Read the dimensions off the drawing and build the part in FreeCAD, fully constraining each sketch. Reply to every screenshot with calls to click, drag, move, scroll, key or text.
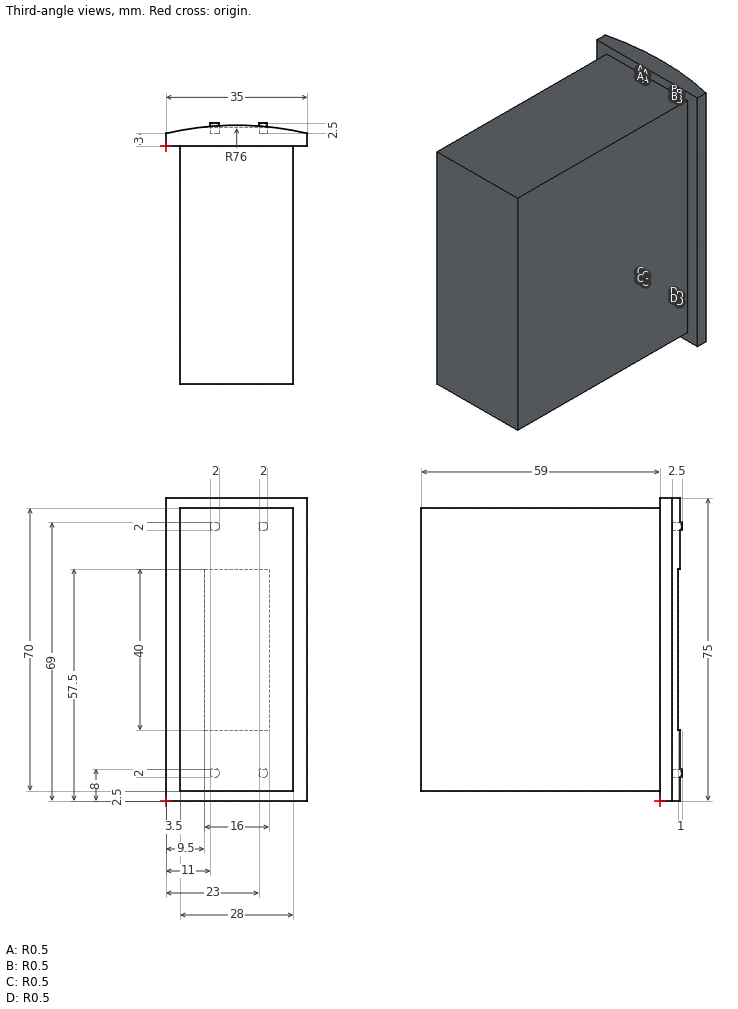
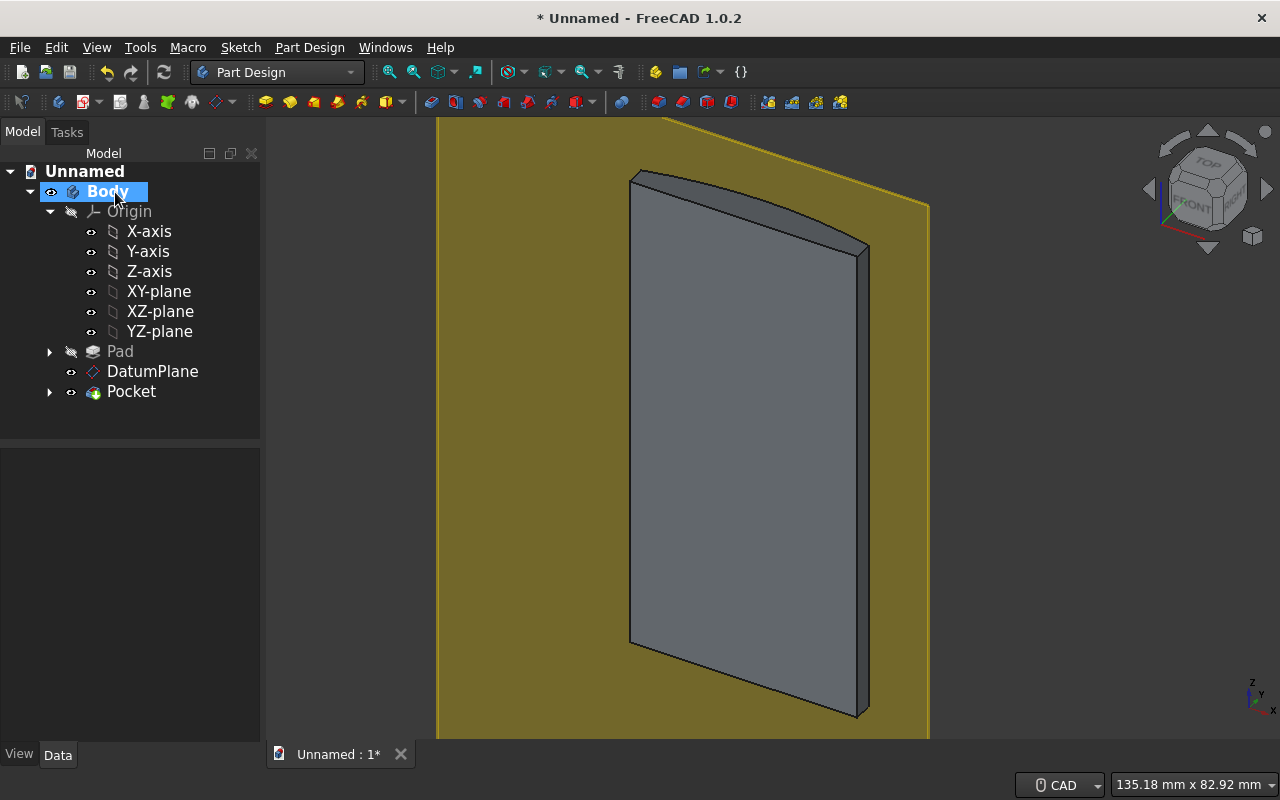
click(116, 372)
key(space)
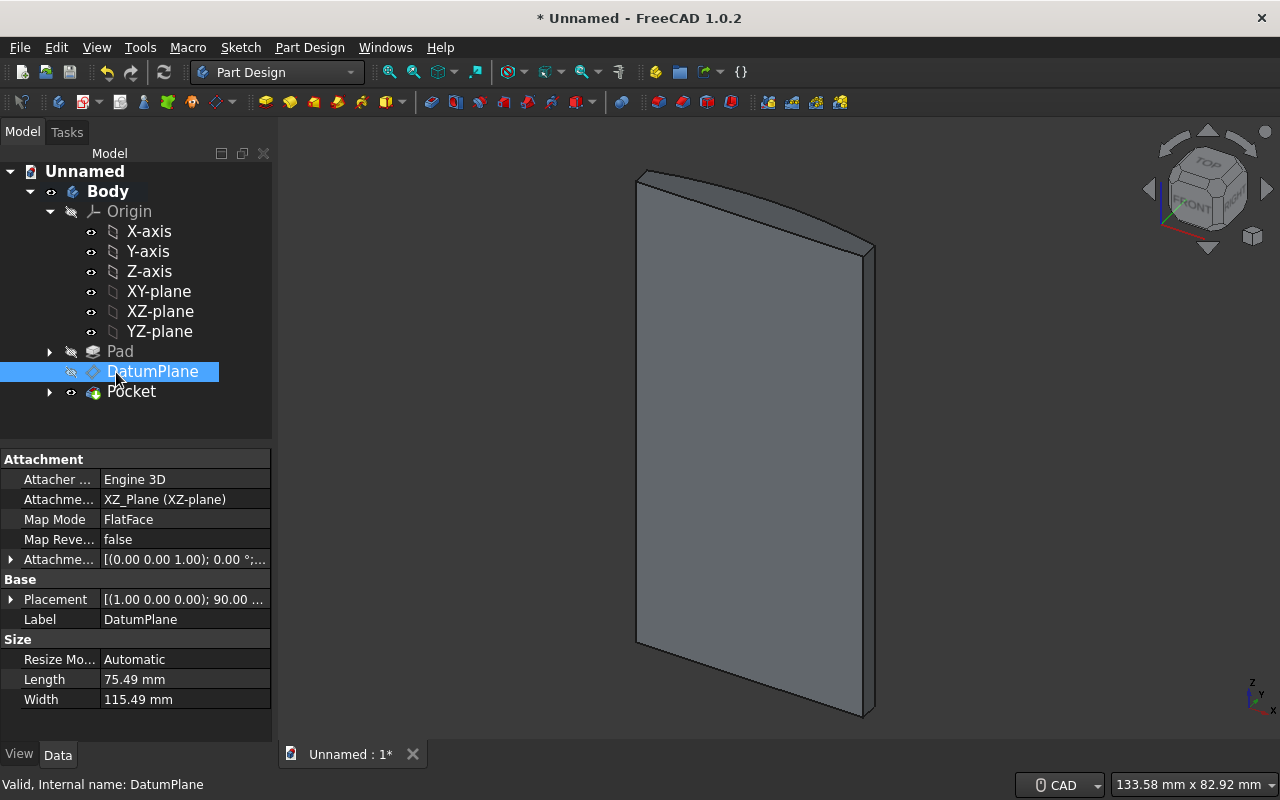
click(318, 699)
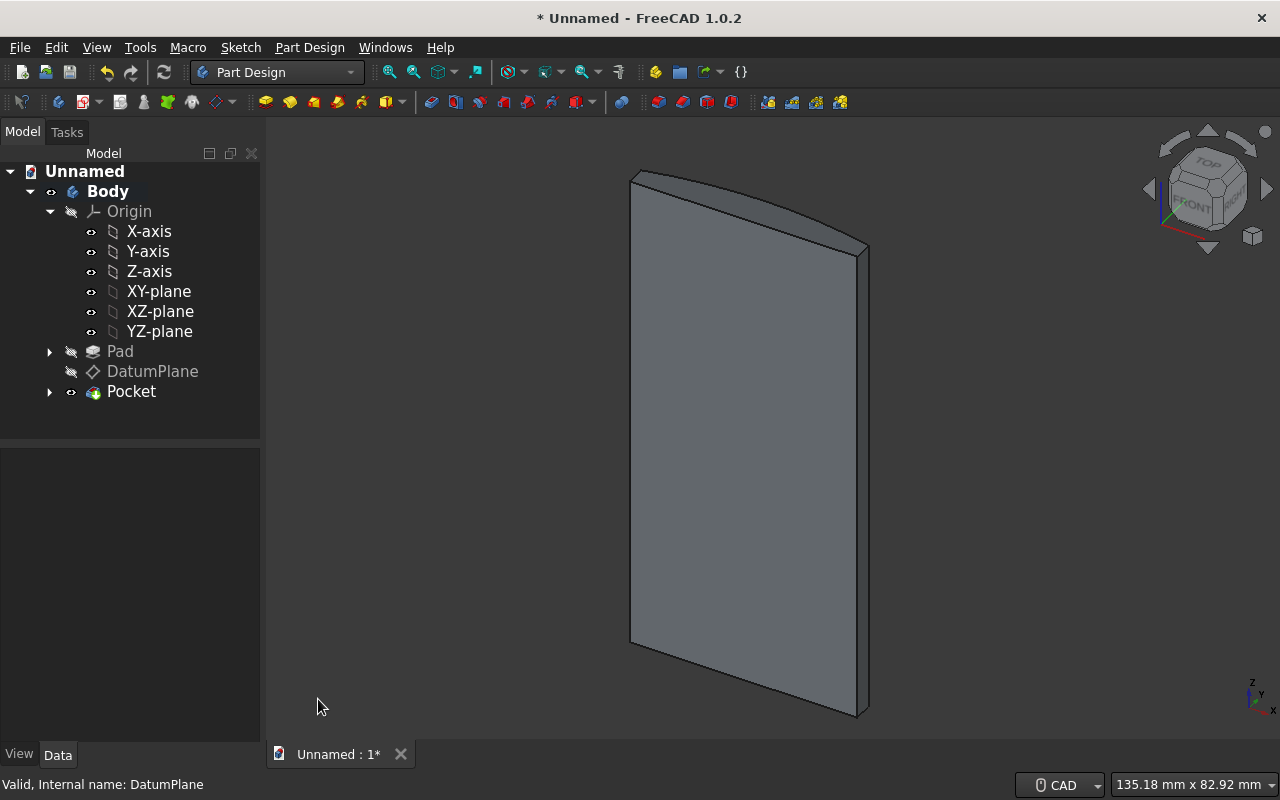
click(84, 102)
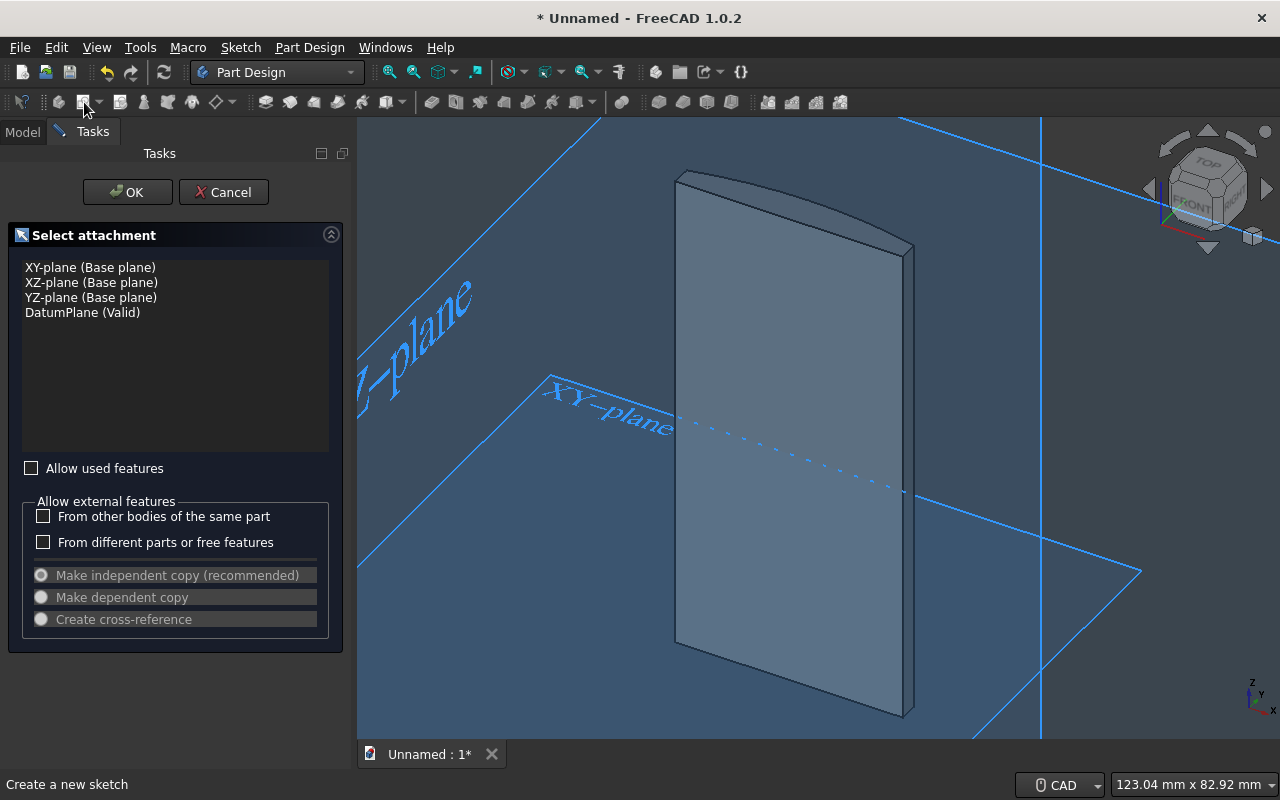
click(82, 282)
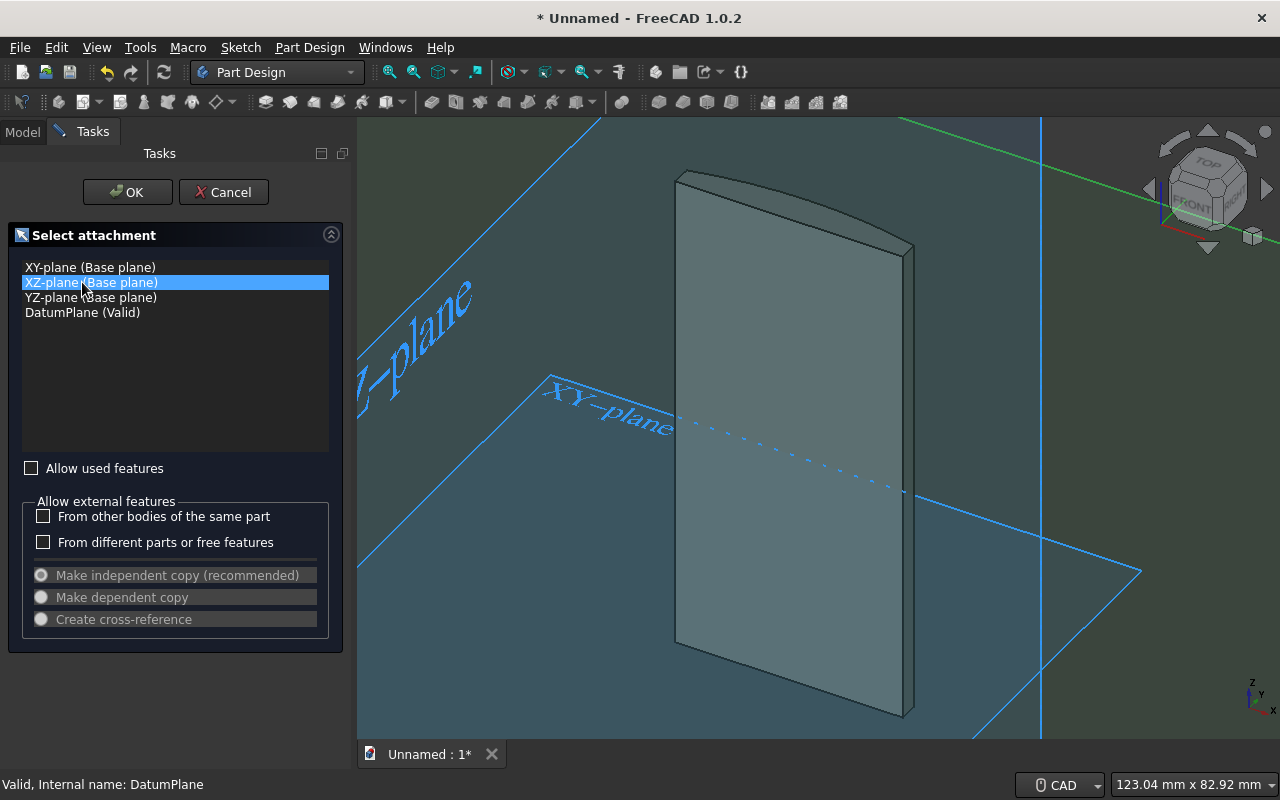
click(128, 192)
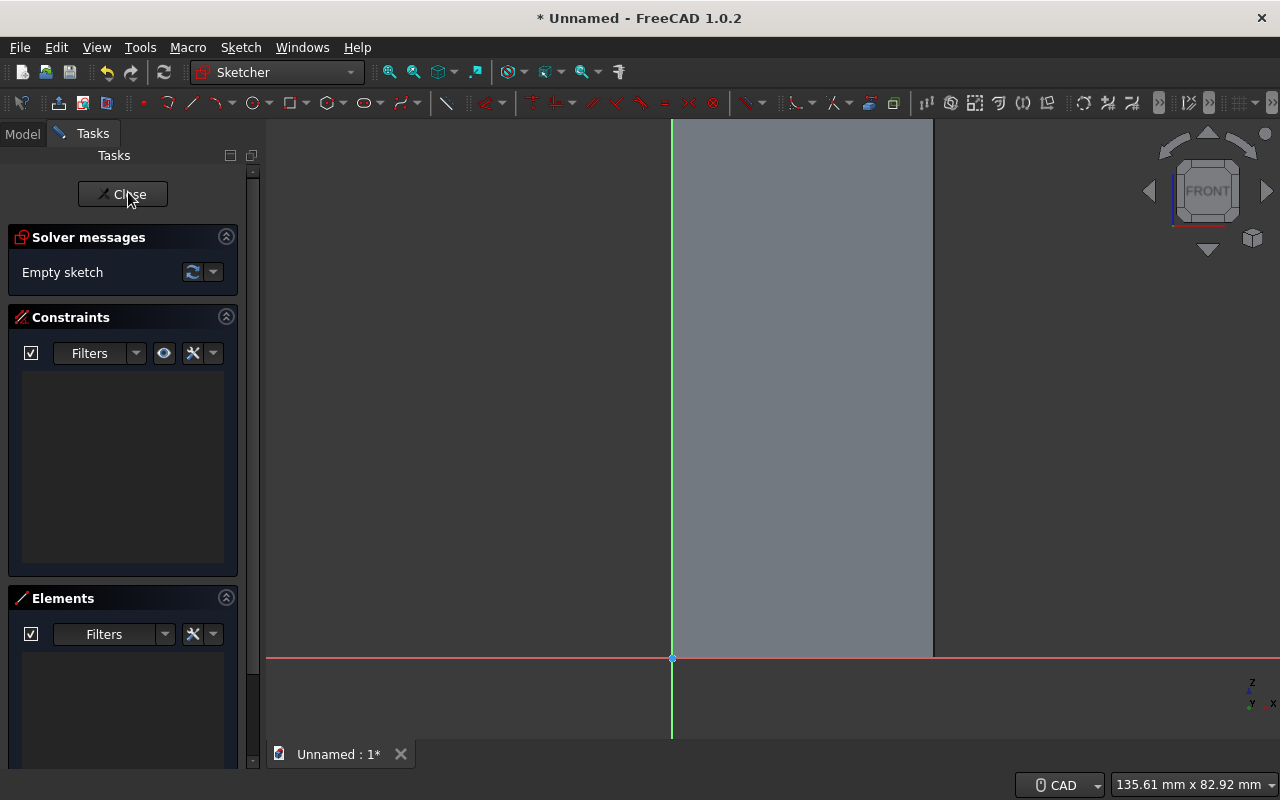
scroll(531, 514, down, 2)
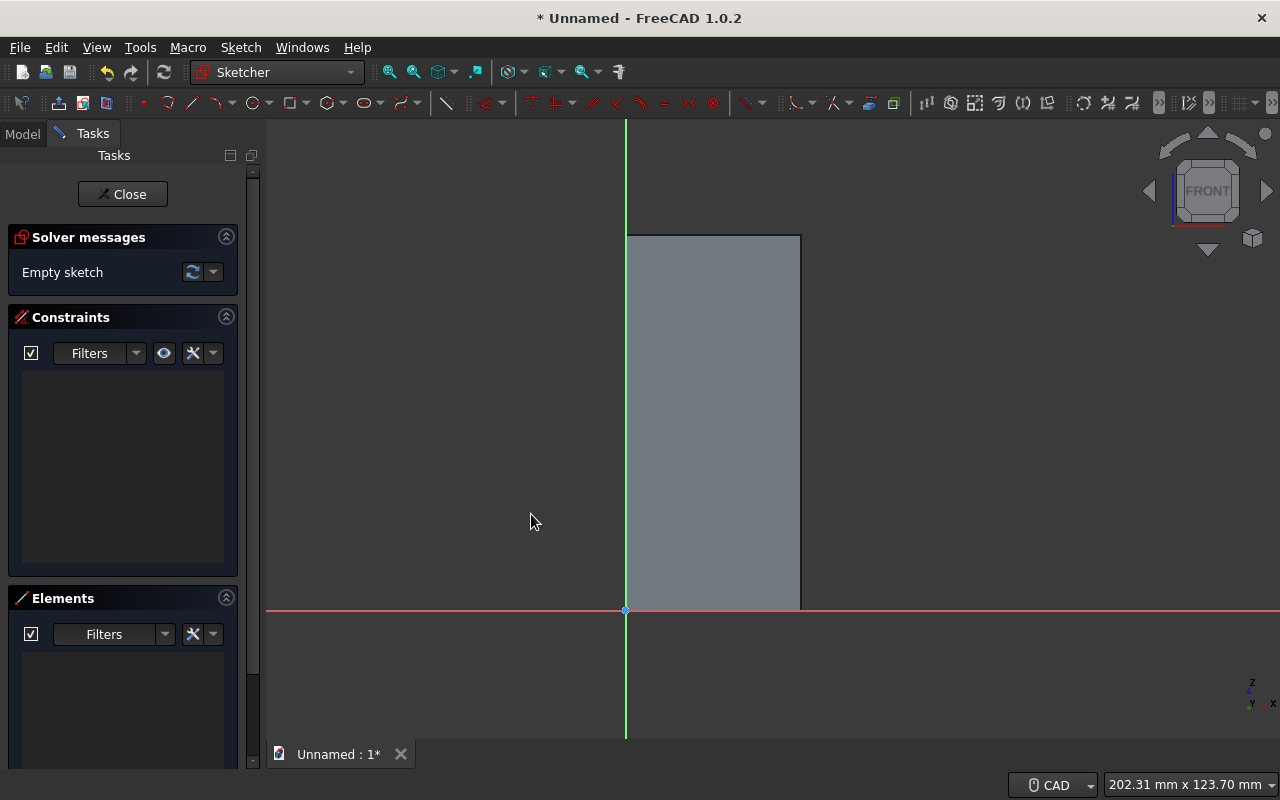
key(g)
key(r)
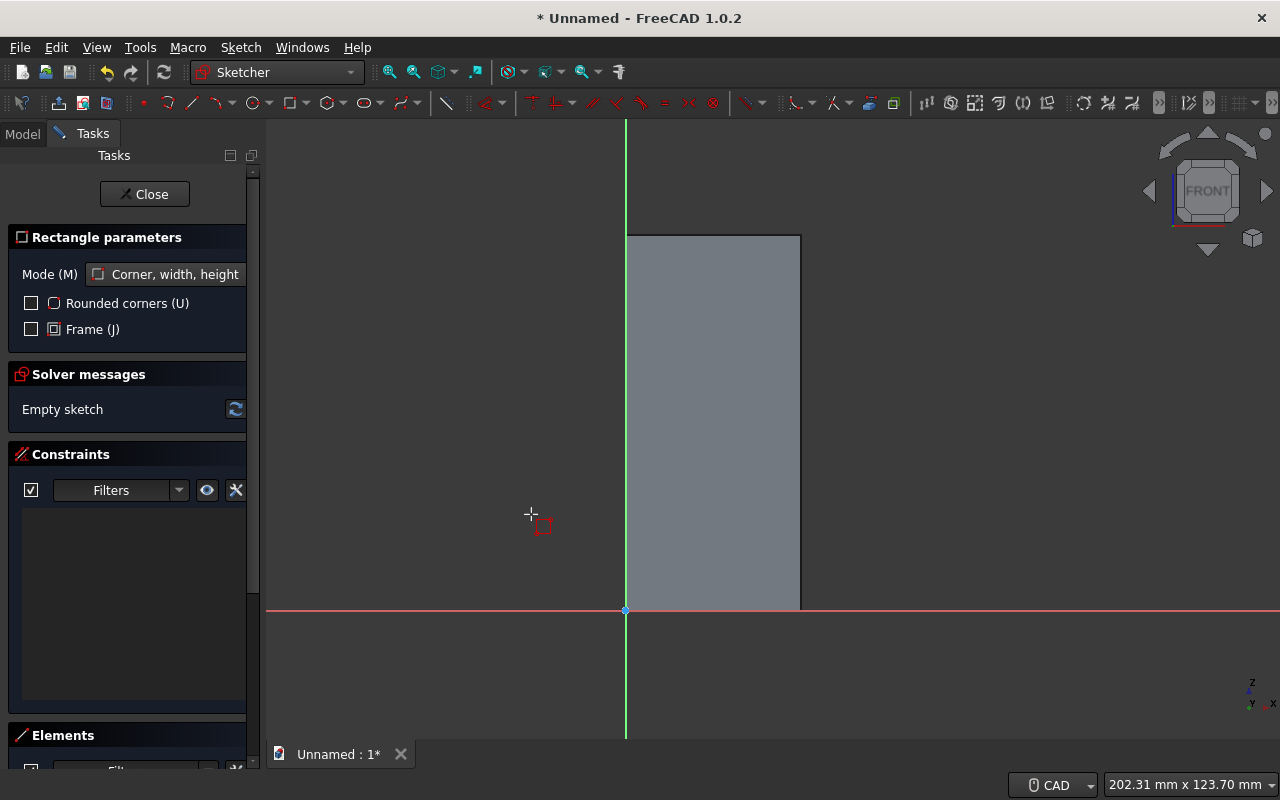
click(643, 247)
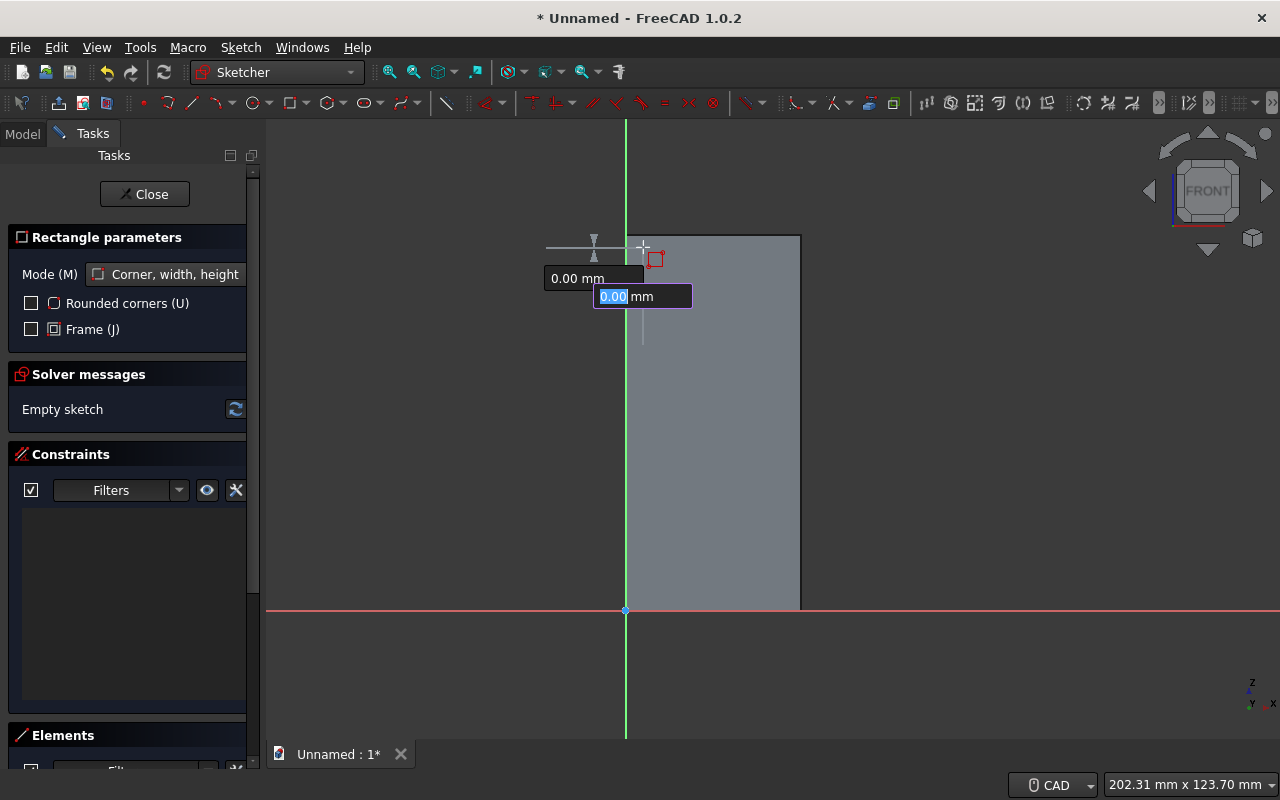
scroll(784, 598, up, 2)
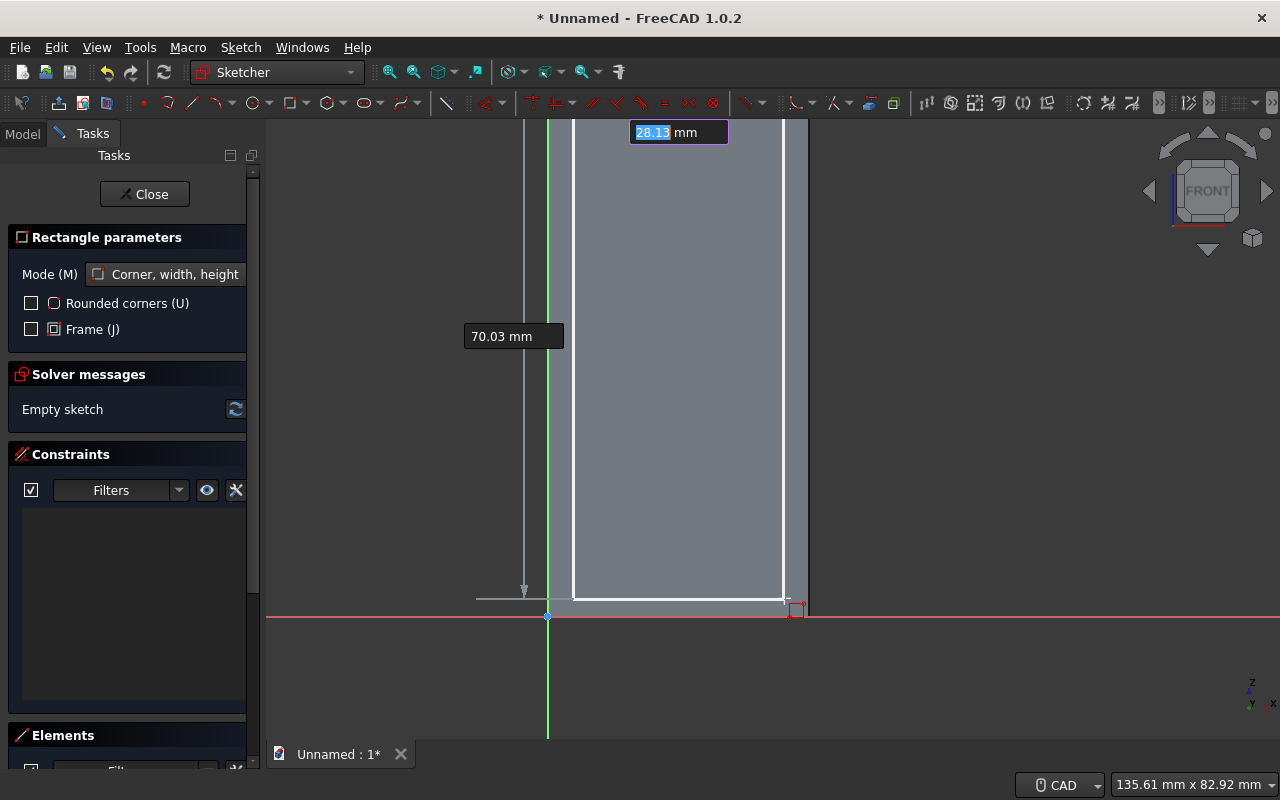
click(783, 598)
key(Escape)